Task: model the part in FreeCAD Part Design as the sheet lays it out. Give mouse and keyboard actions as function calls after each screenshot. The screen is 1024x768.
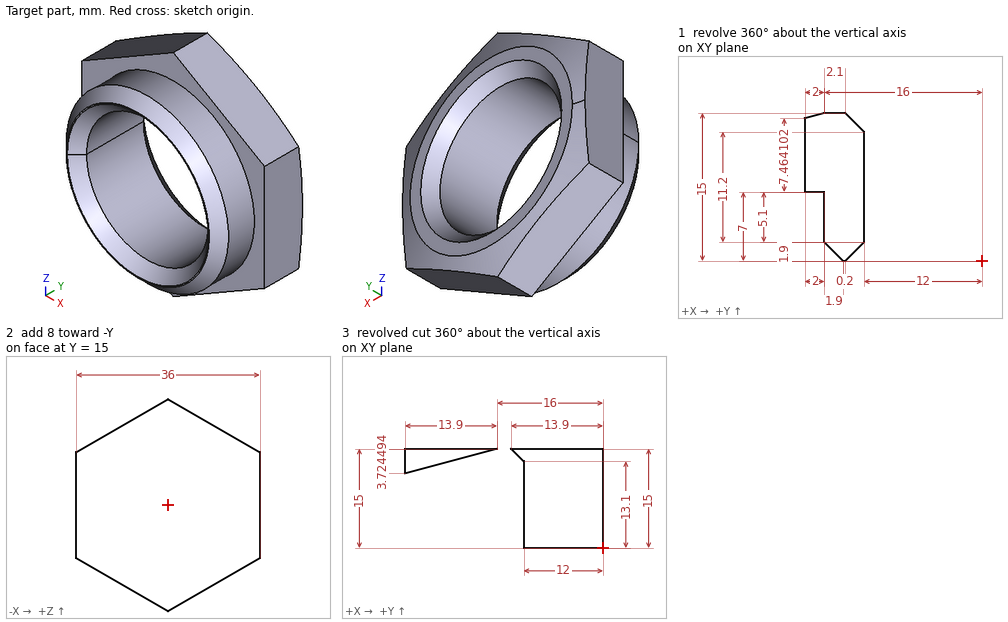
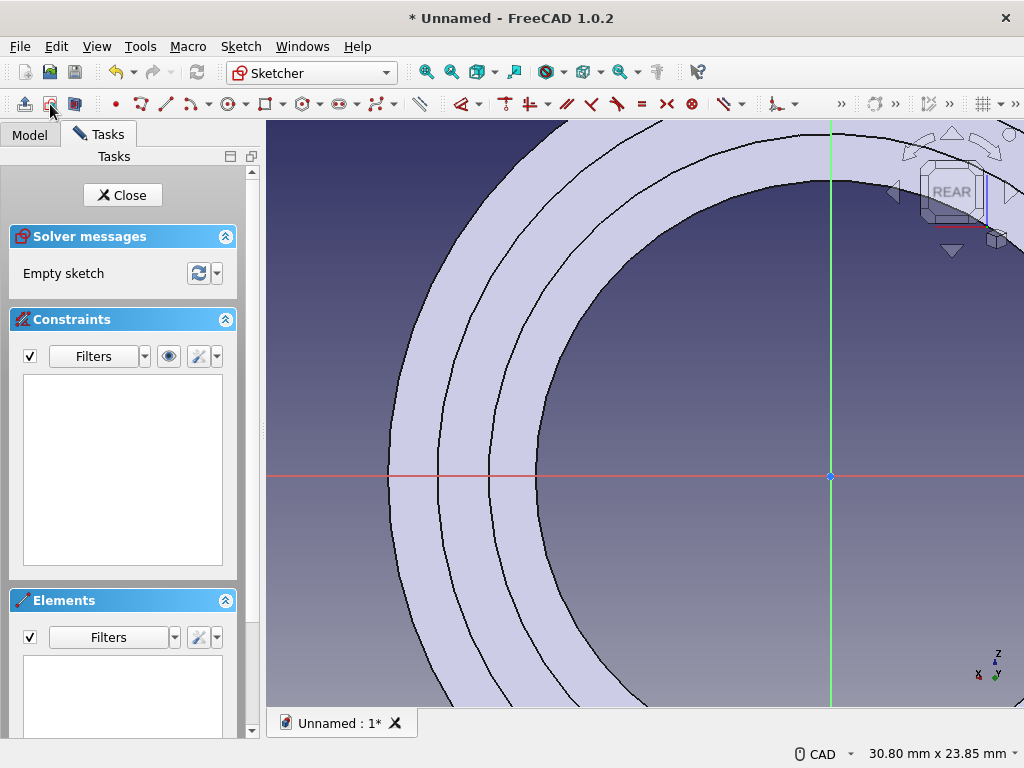
scroll(428, 377, down, 5)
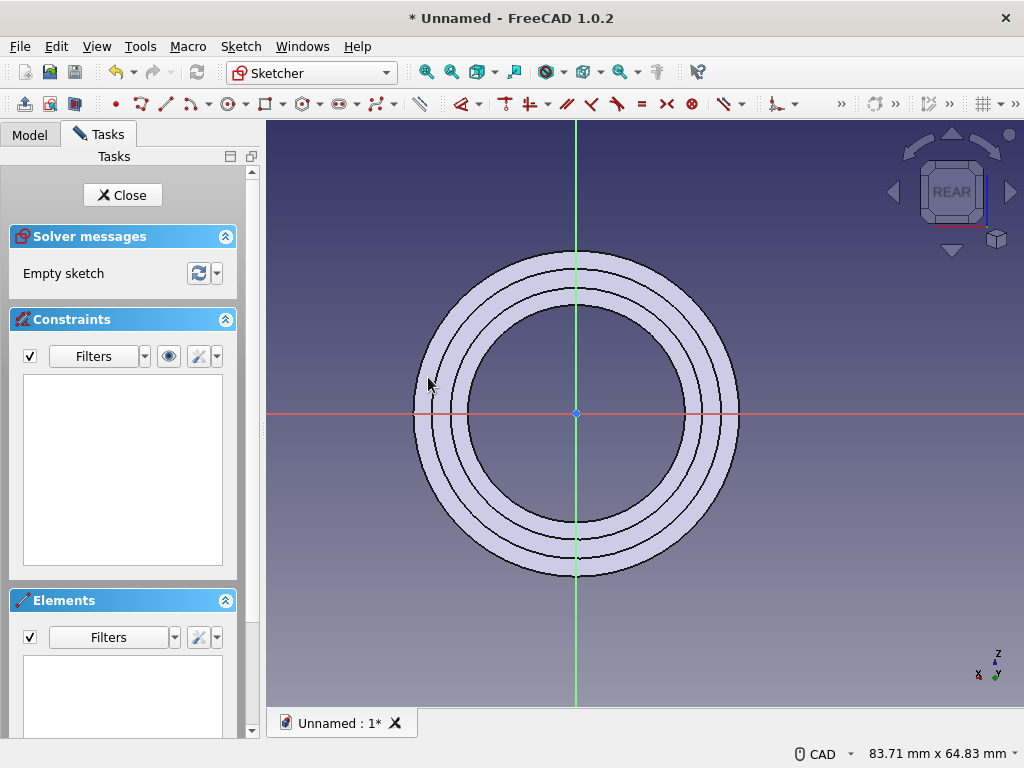
key(g)
key(p)
key(6)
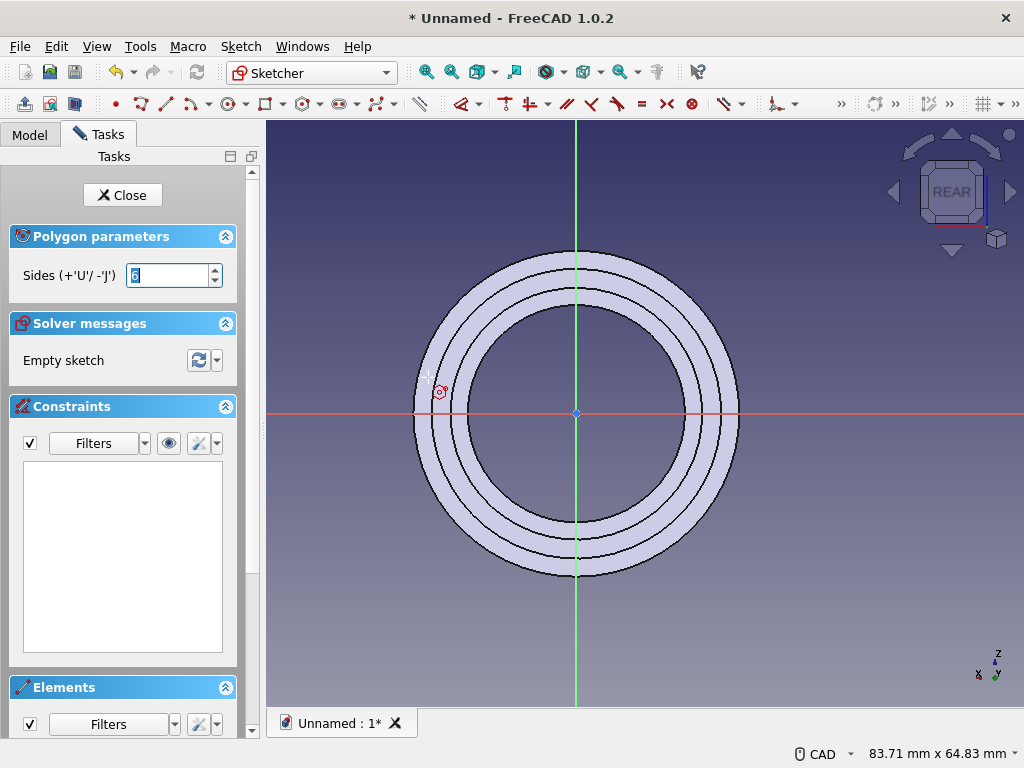
click(576, 414)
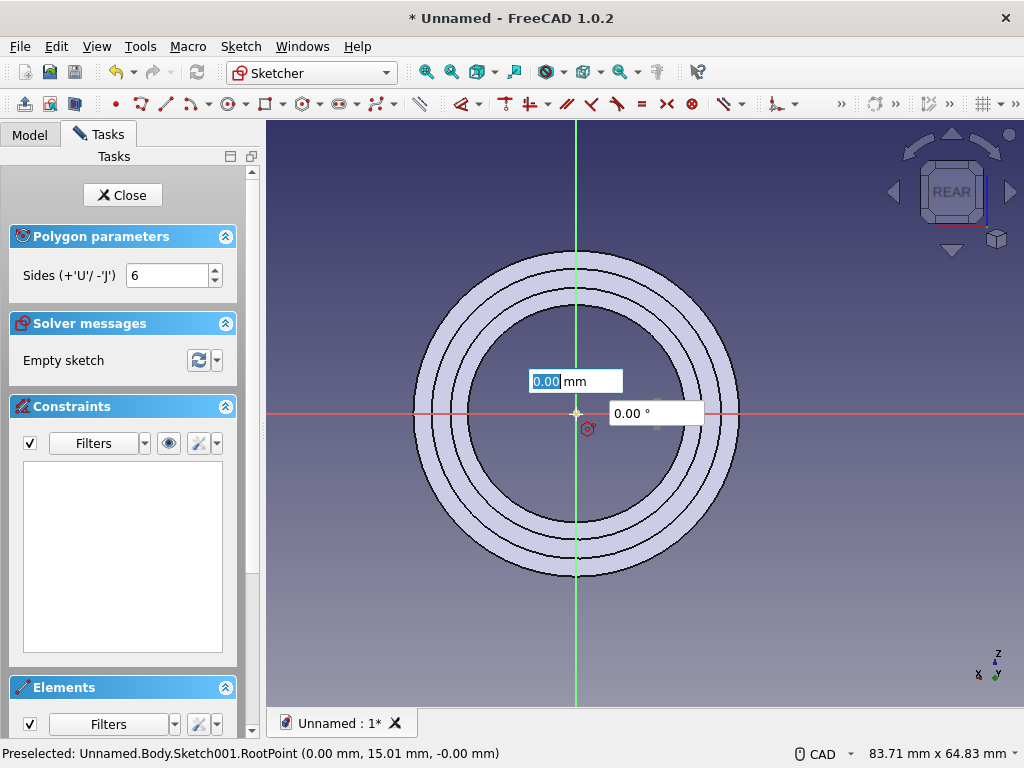
click(576, 602)
right_click(576, 602)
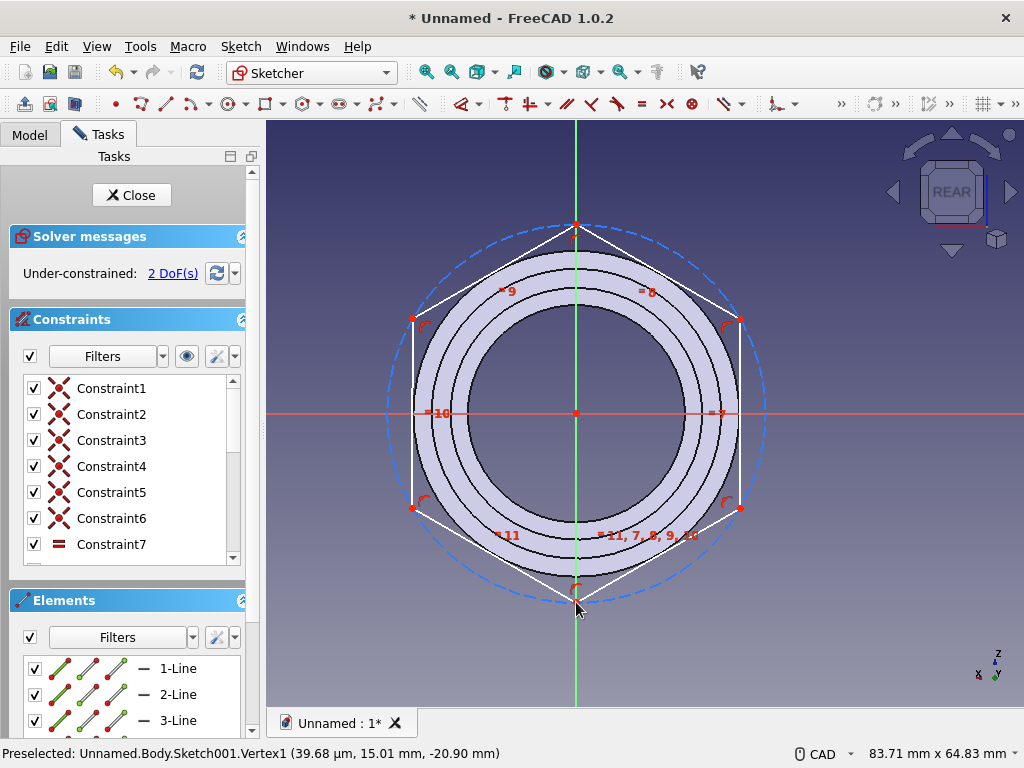
click(740, 452)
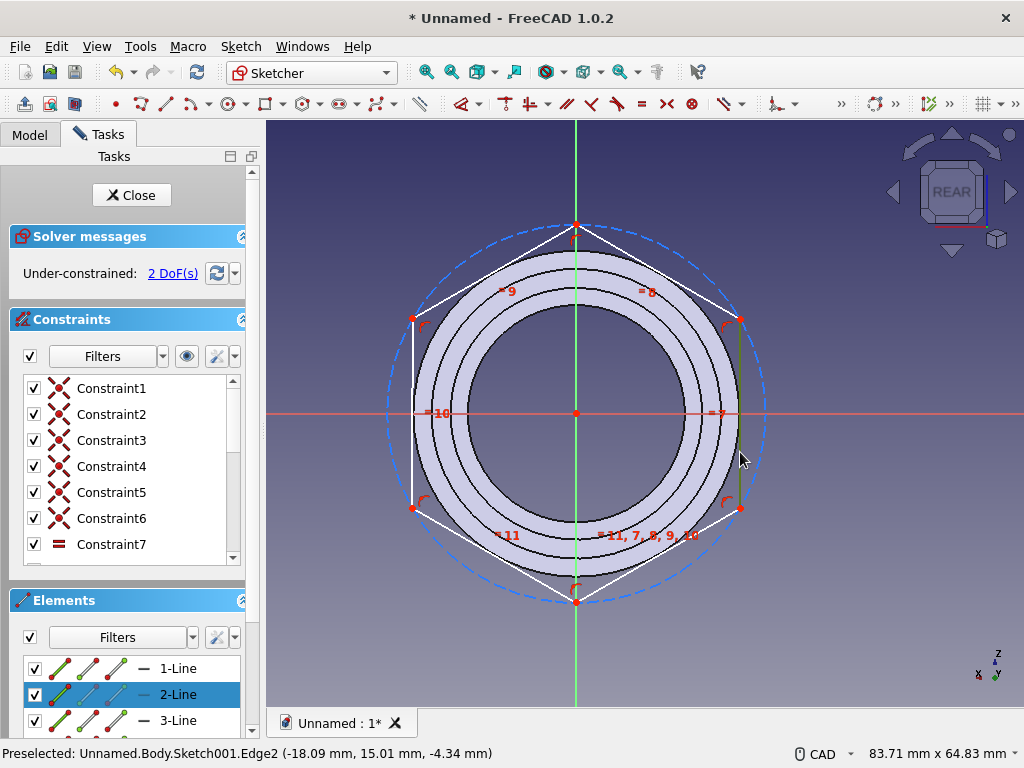
key(v)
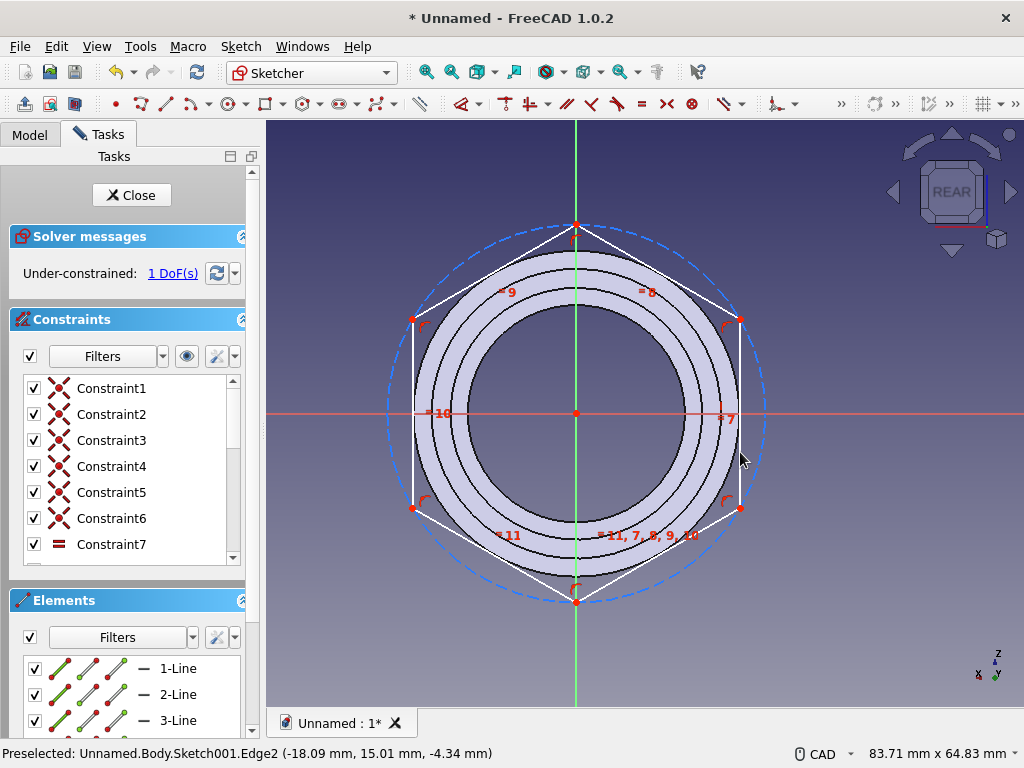
key(d)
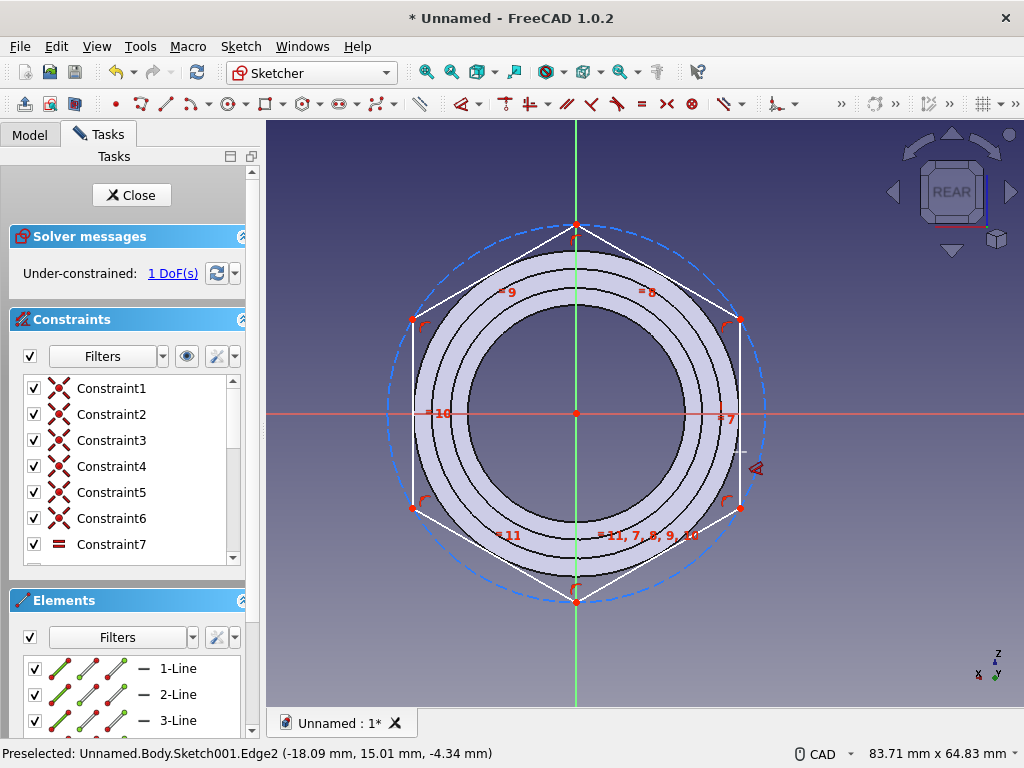
click(413, 319)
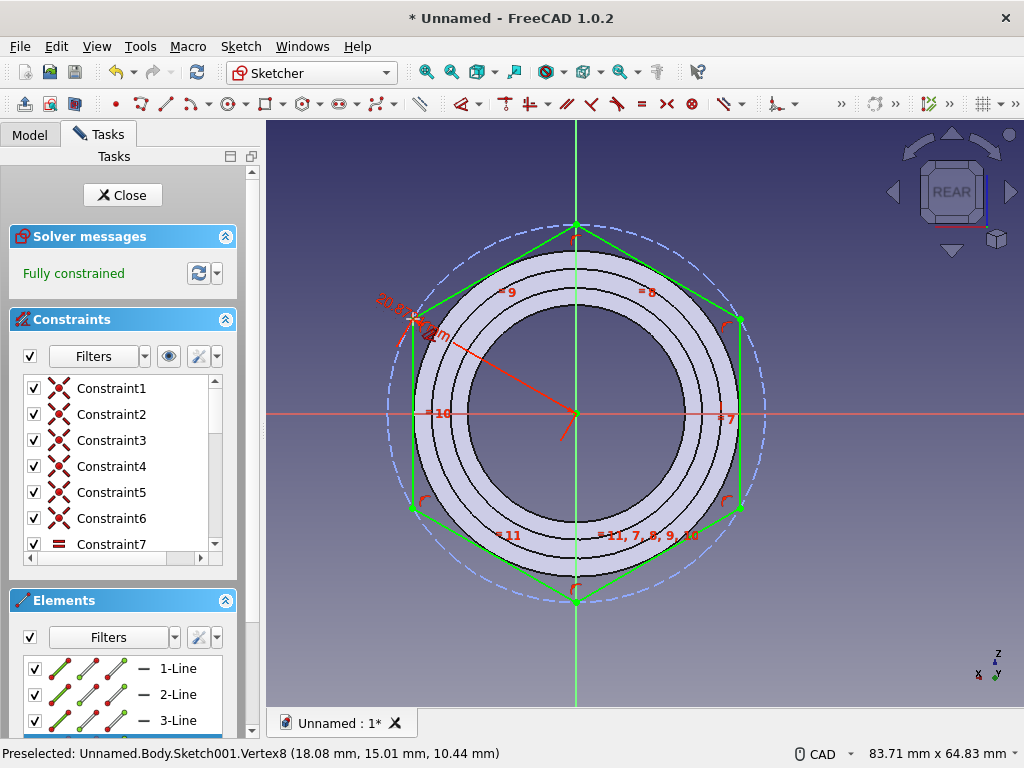
click(740, 508)
click(501, 542)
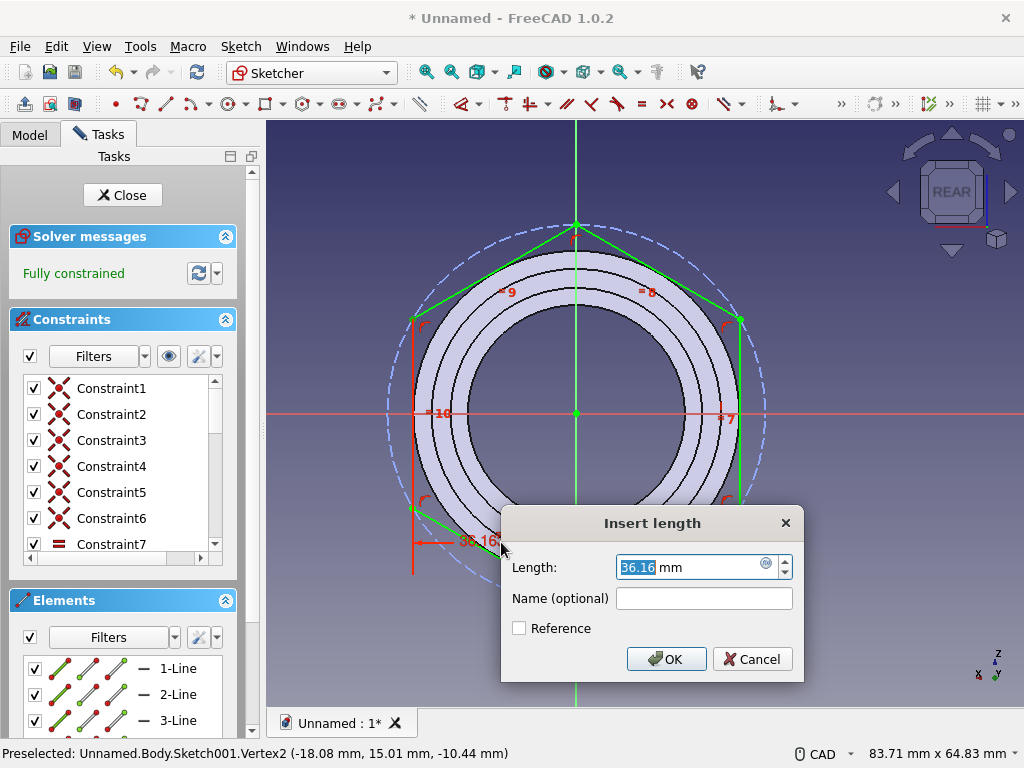
text(36)
key(Return)
key(Escape)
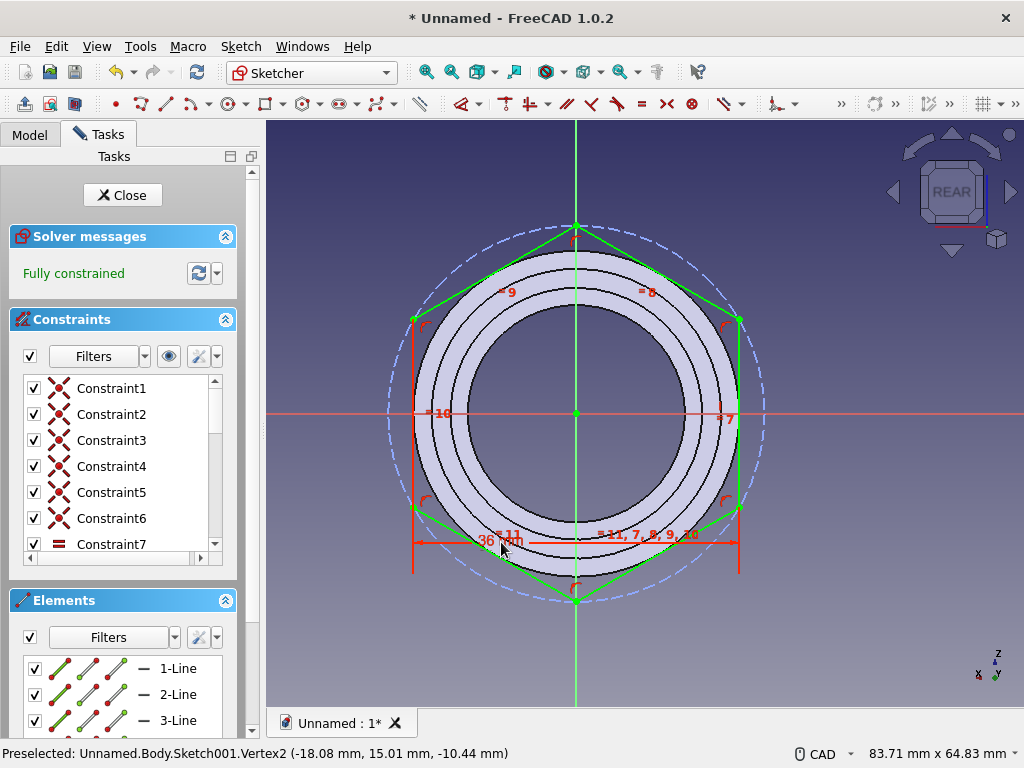
click(123, 195)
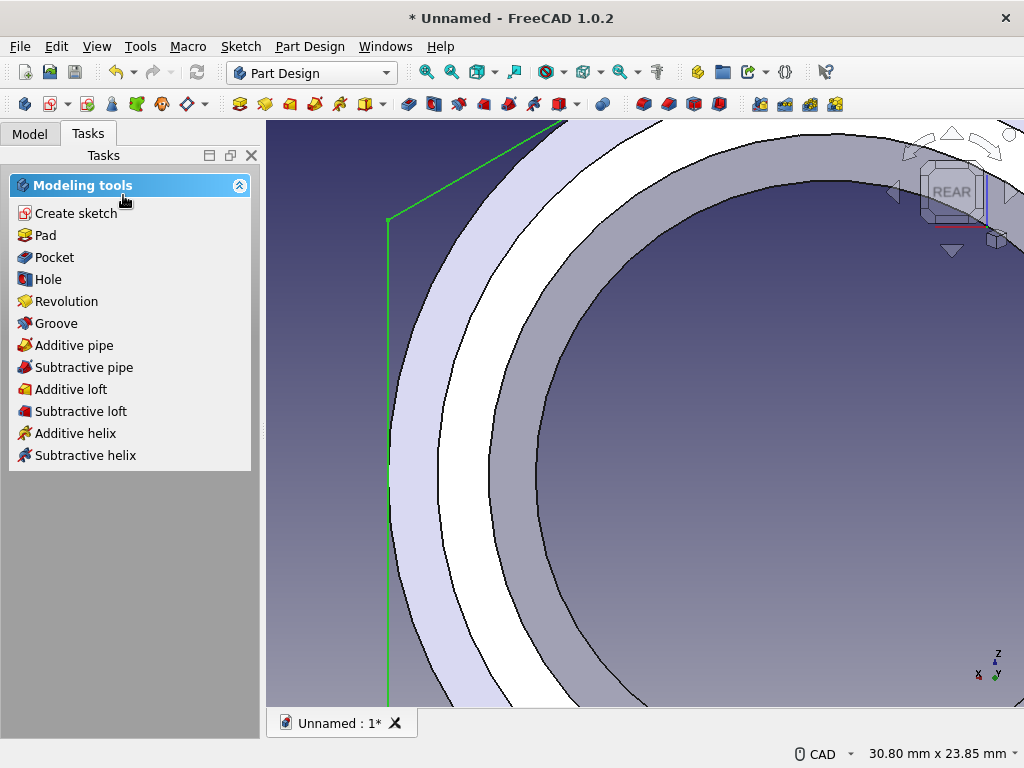
click(240, 104)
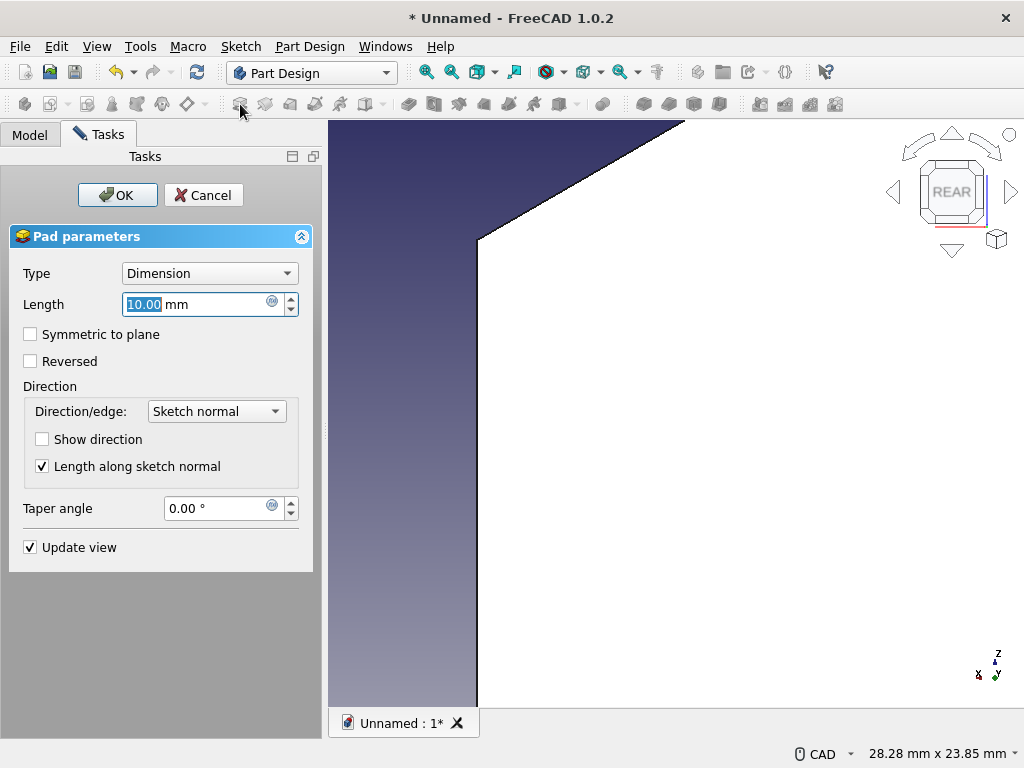
text(8)
key(Tab)